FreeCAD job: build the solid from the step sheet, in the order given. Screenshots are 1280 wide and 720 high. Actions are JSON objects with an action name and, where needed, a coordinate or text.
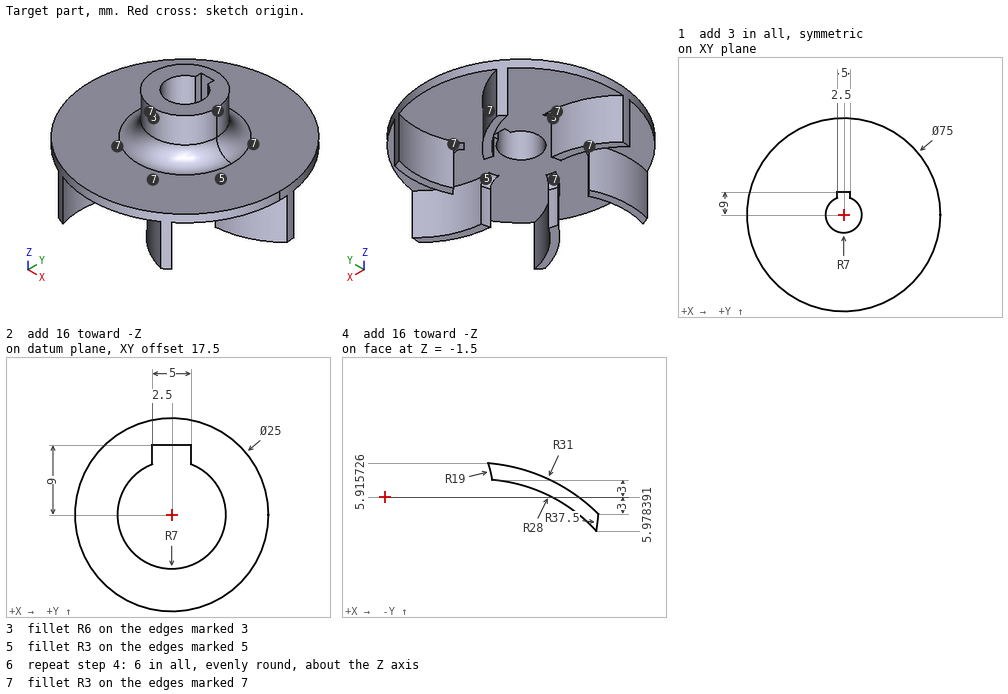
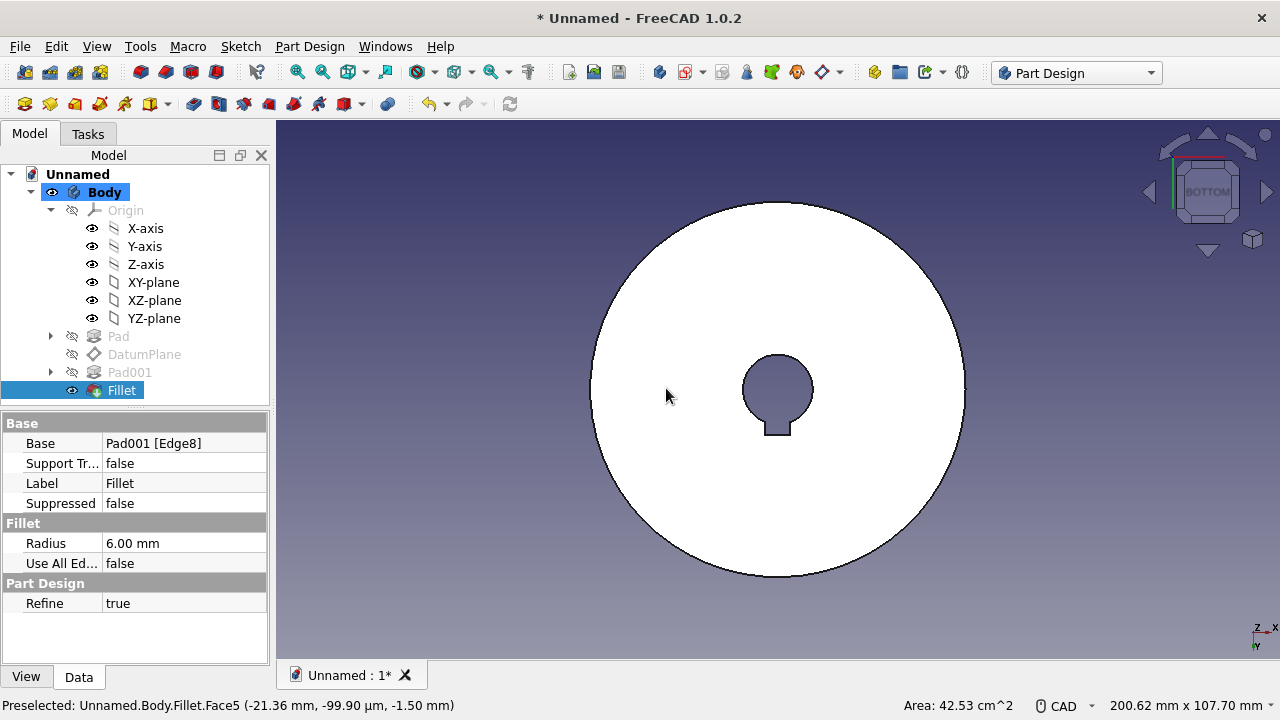
{"action": "left_click", "coordinate": [684, 72]}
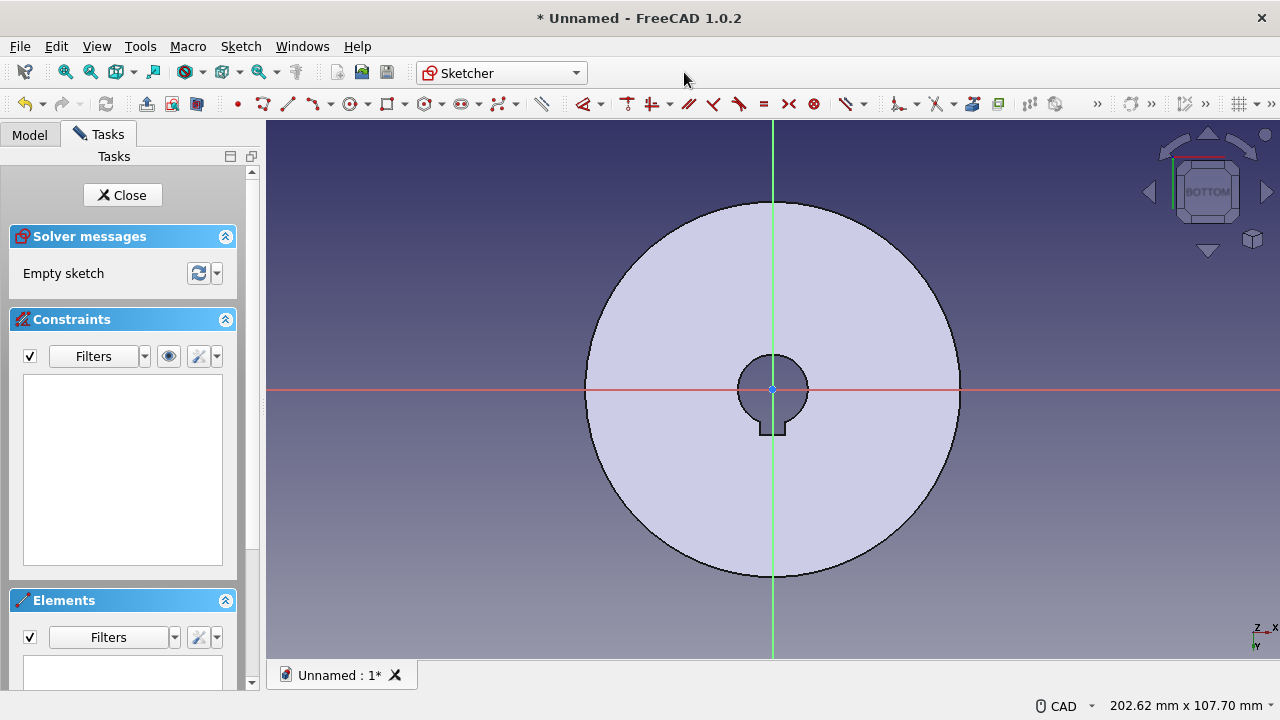
{"action": "scroll", "coordinate": [936, 390], "scroll_direction": "up", "scroll_amount": 6}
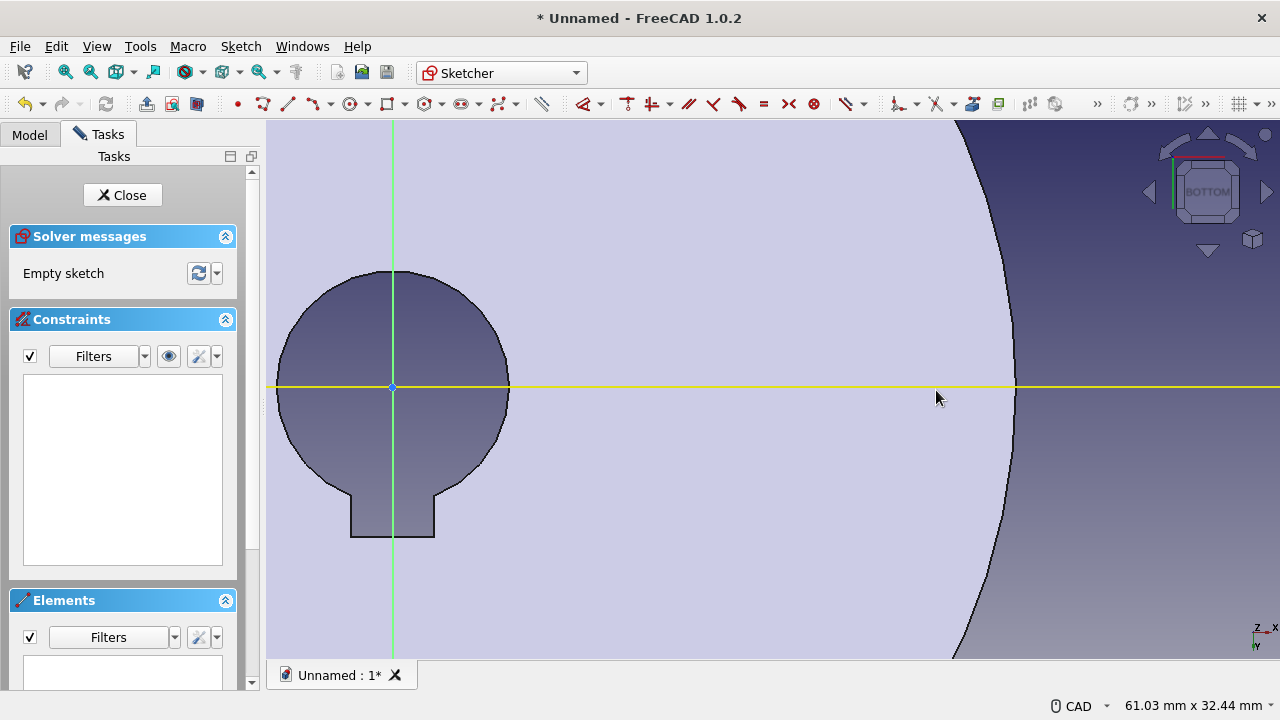
{"action": "left_click", "coordinate": [312, 104]}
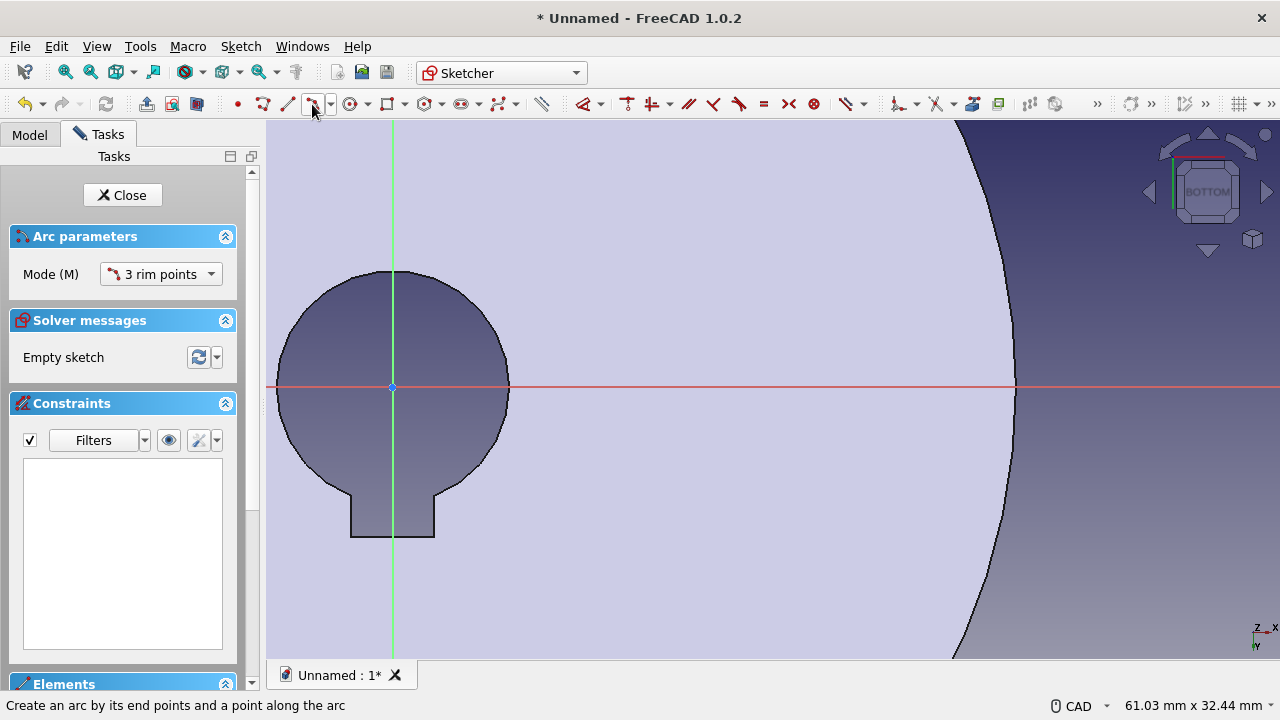
{"action": "left_click", "coordinate": [705, 337]}
{"action": "left_click", "coordinate": [1008, 487]}
{"action": "left_click", "coordinate": [839, 369]}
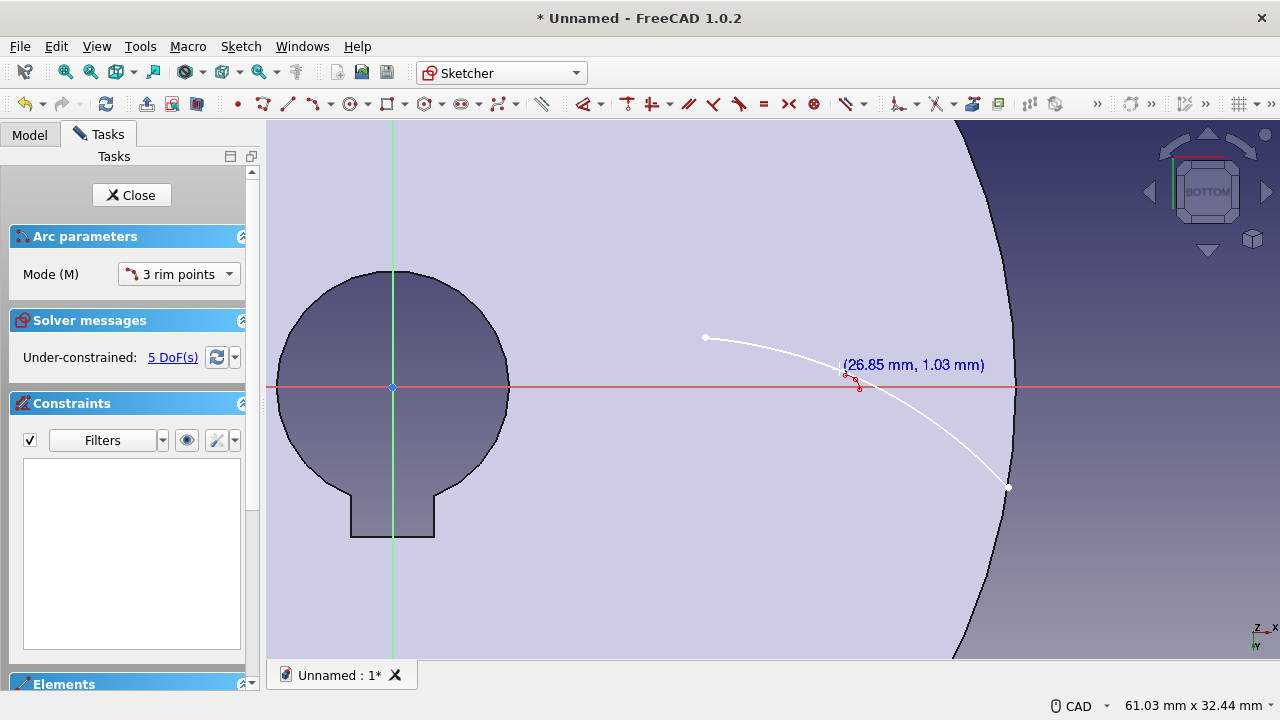
{"action": "left_click", "coordinate": [1008, 488]}
{"action": "left_click", "coordinate": [1014, 437]}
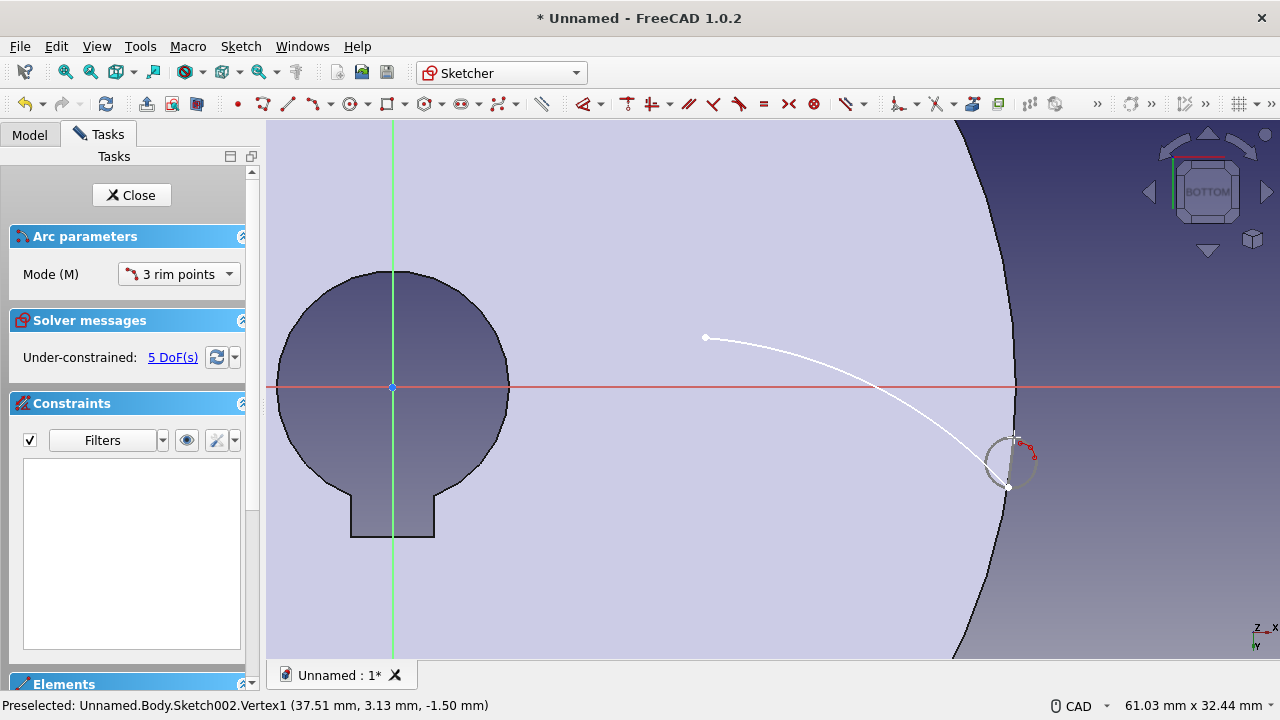
{"action": "scroll", "coordinate": [1011, 462], "scroll_direction": "up", "scroll_amount": 18}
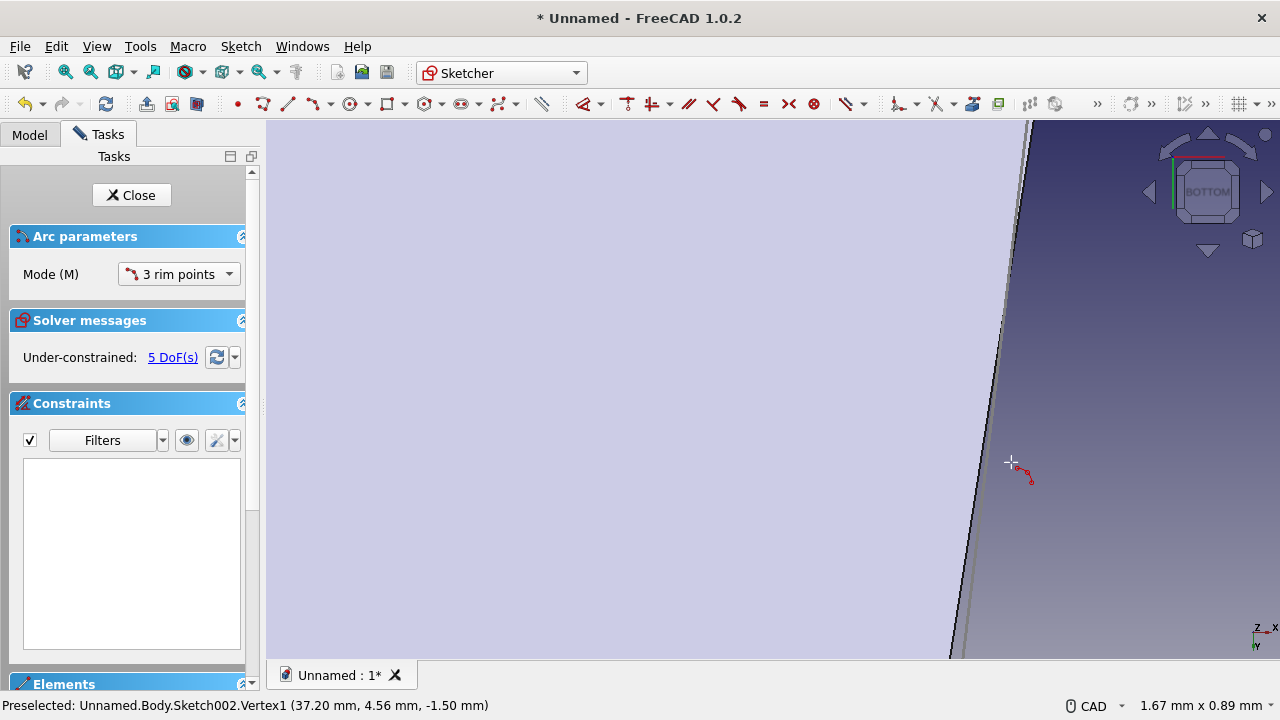
{"action": "left_click", "coordinate": [1002, 433]}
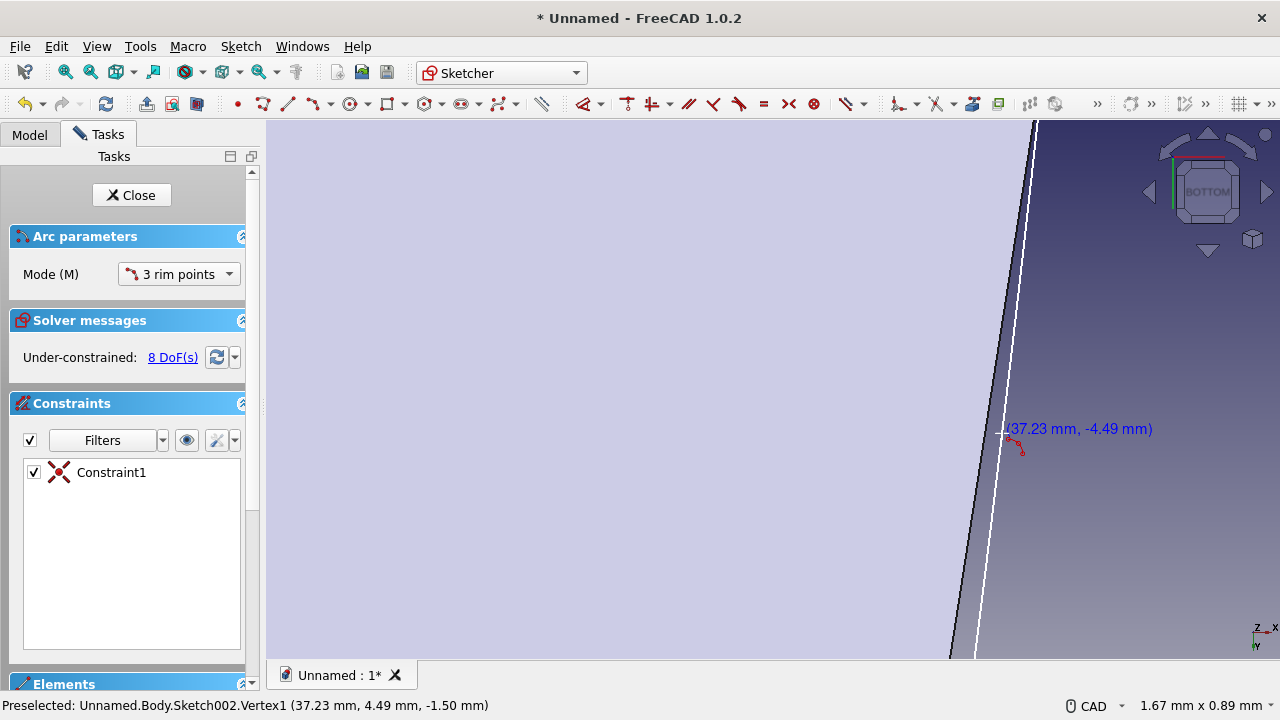
{"action": "scroll", "coordinate": [1083, 482], "scroll_direction": "down", "scroll_amount": 17}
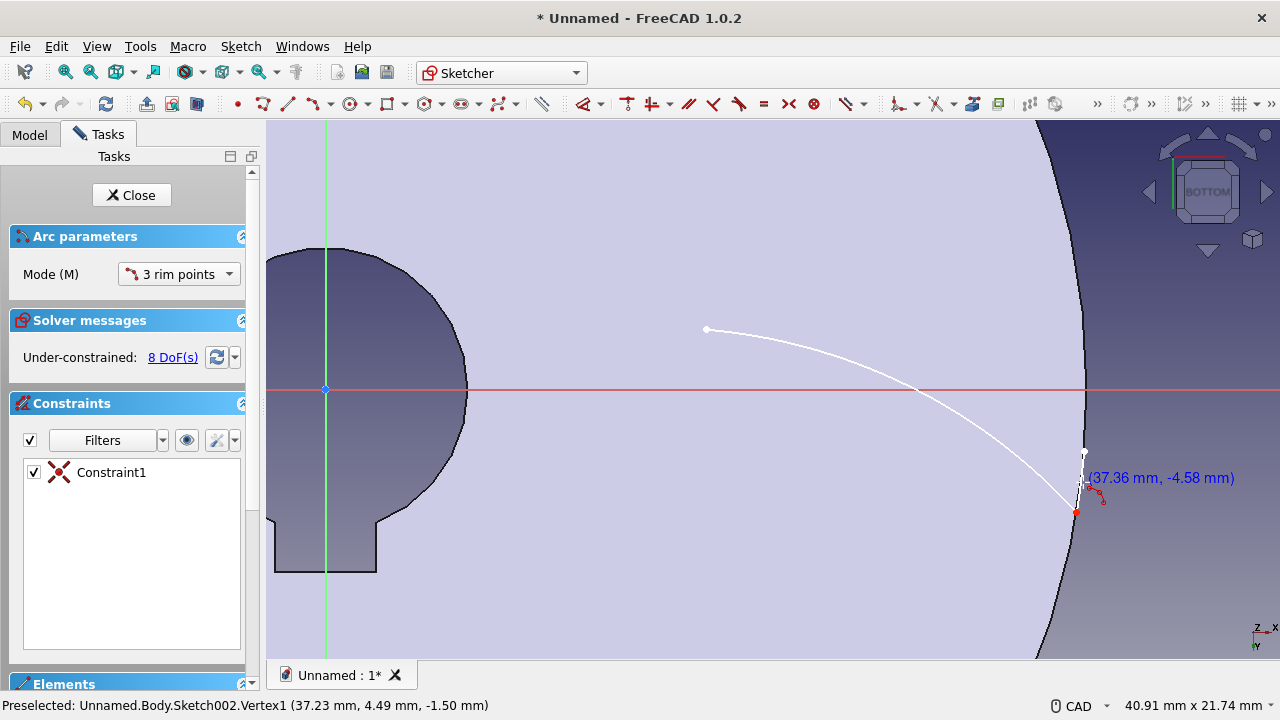
{"action": "left_click", "coordinate": [1084, 452]}
{"action": "left_click", "coordinate": [692, 270]}
{"action": "left_click", "coordinate": [904, 326]}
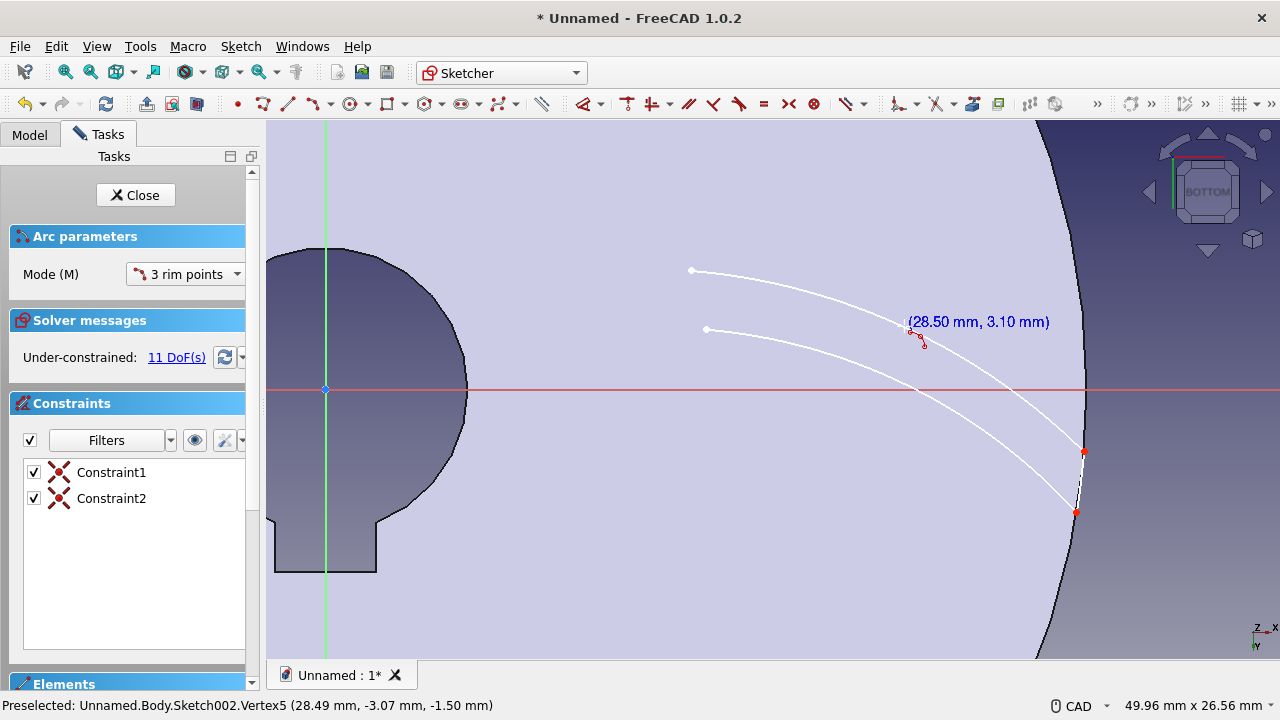
{"action": "left_click", "coordinate": [692, 271]}
{"action": "left_click", "coordinate": [707, 330]}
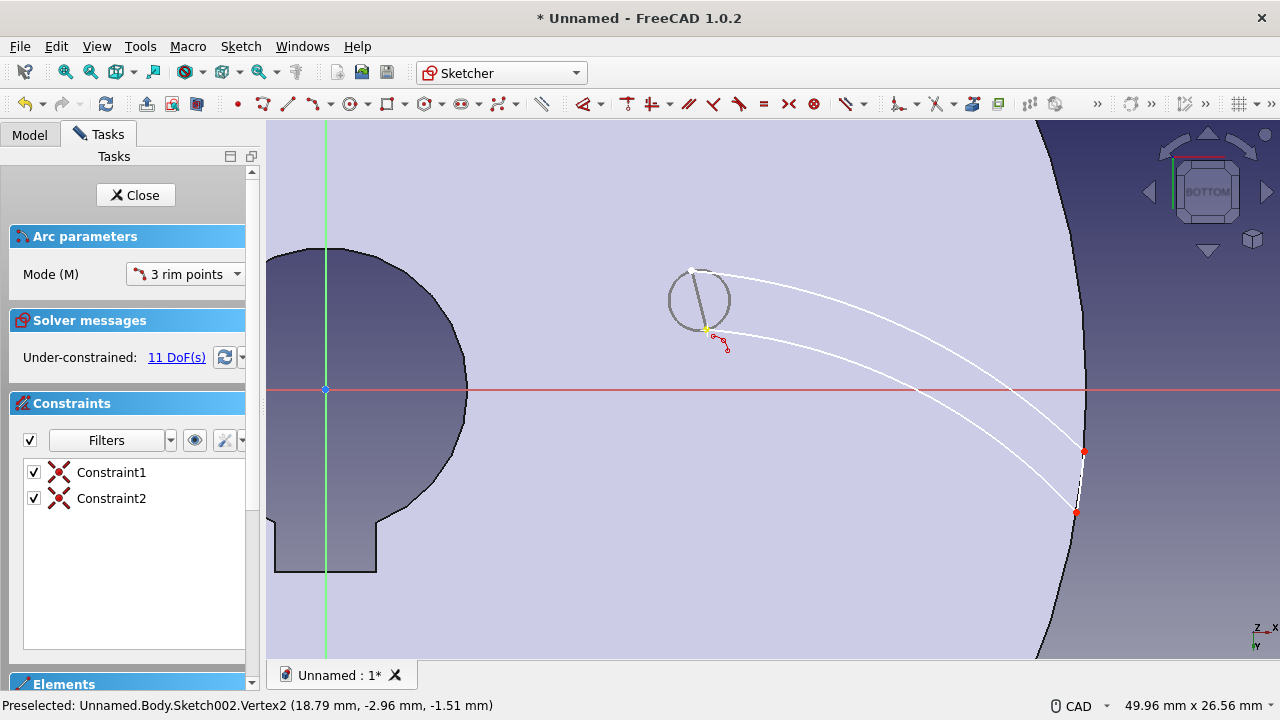
{"action": "scroll", "coordinate": [700, 299], "scroll_direction": "up", "scroll_amount": 13}